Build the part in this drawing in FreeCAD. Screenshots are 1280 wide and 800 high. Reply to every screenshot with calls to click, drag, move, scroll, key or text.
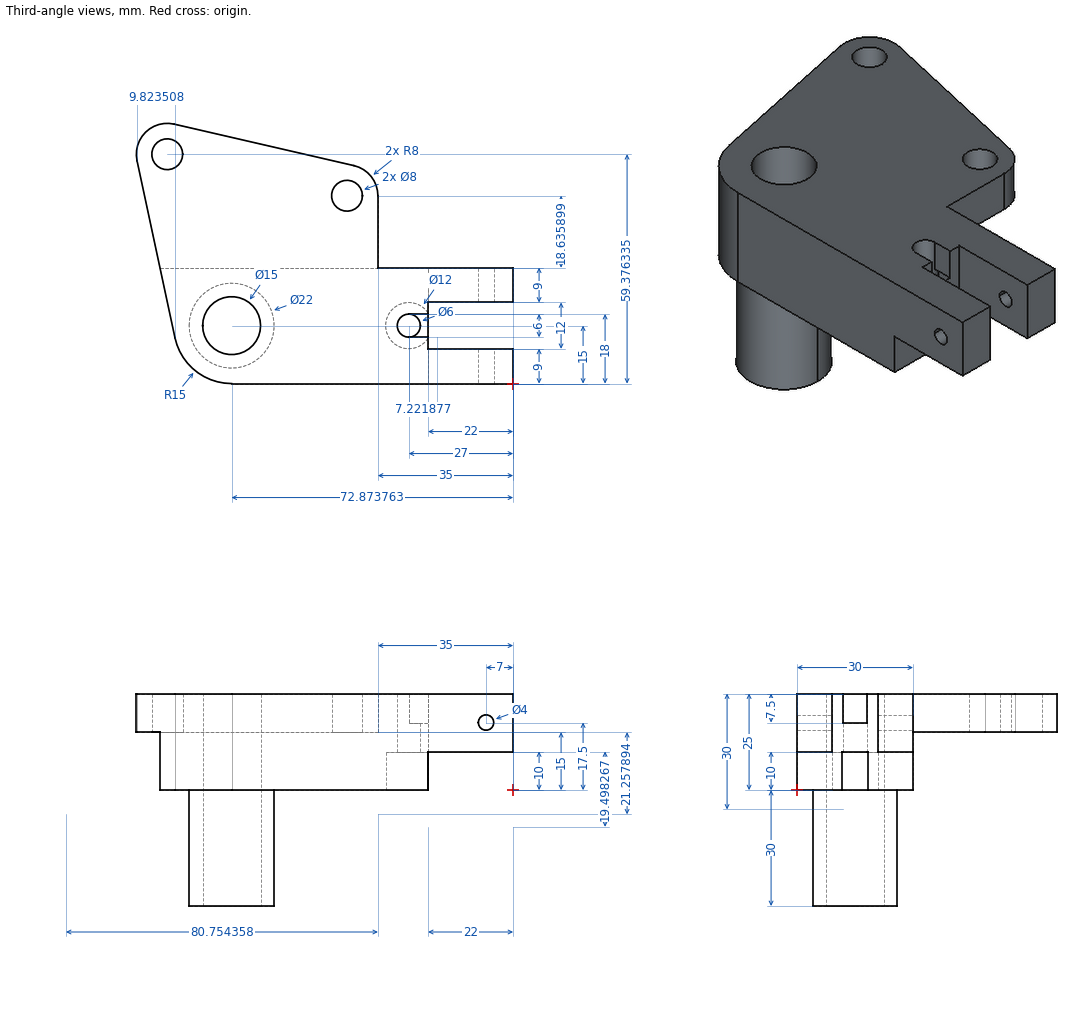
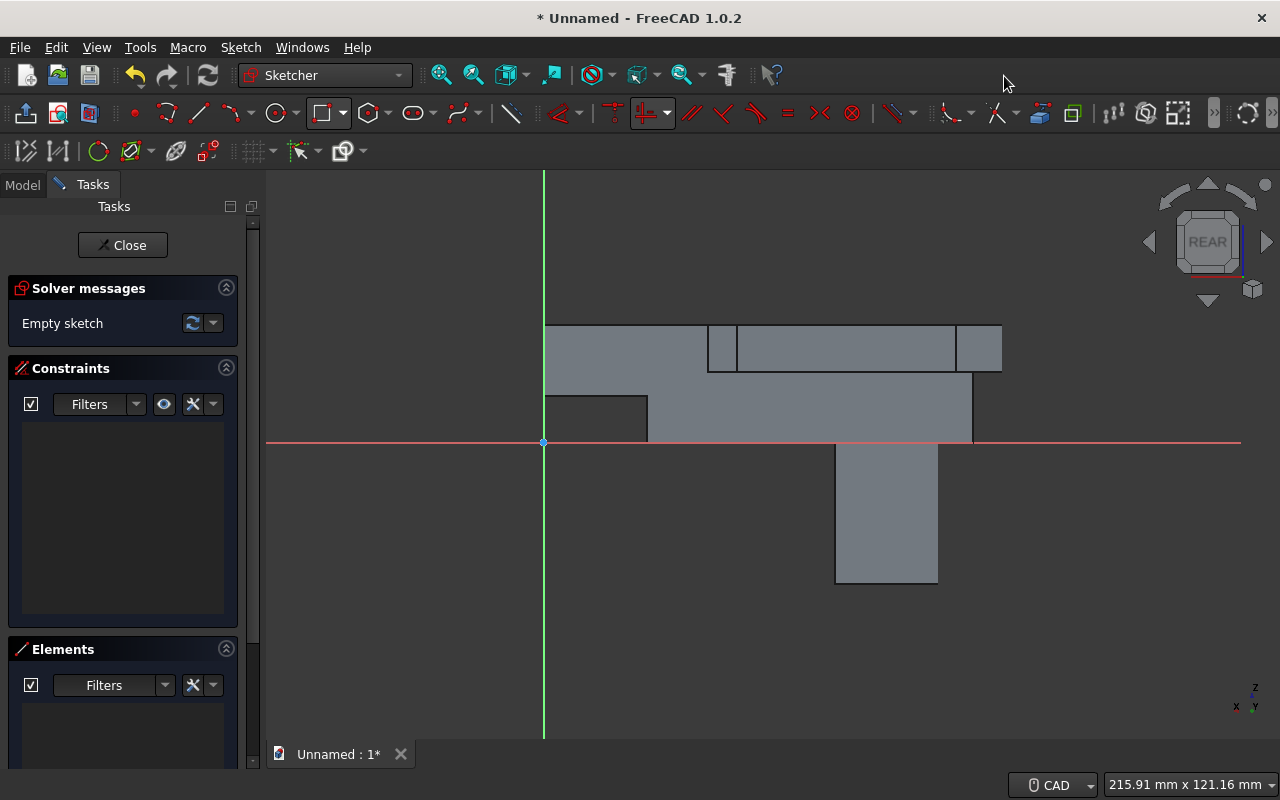
scroll(570, 356, up, 15)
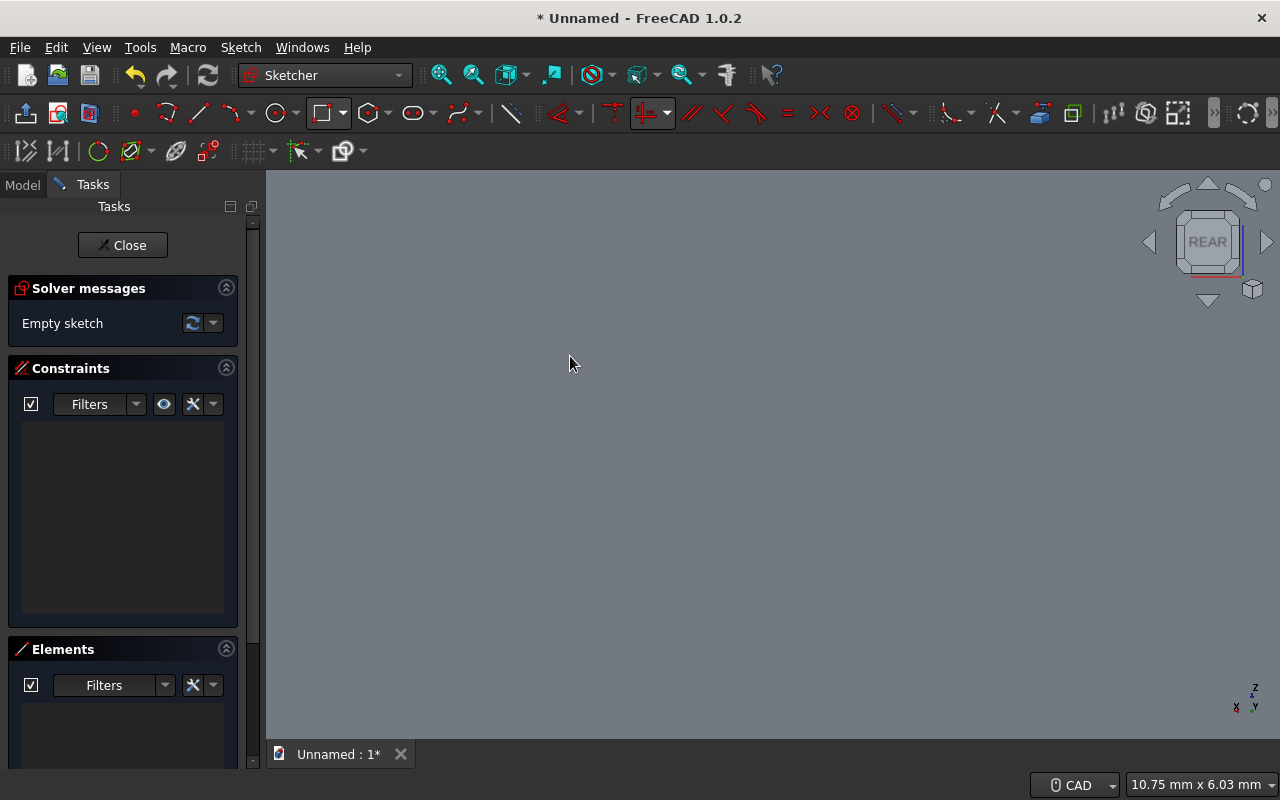
click(276, 114)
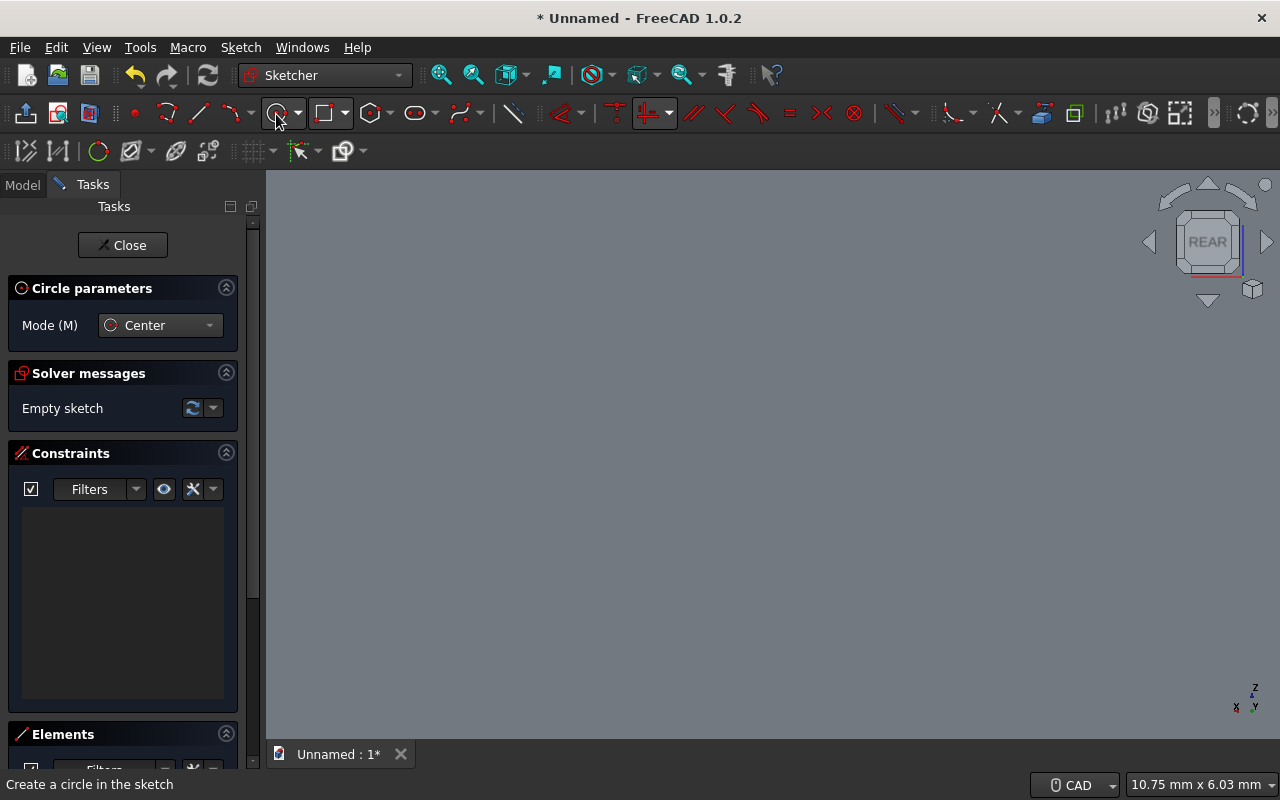
click(701, 442)
click(835, 308)
key(Escape)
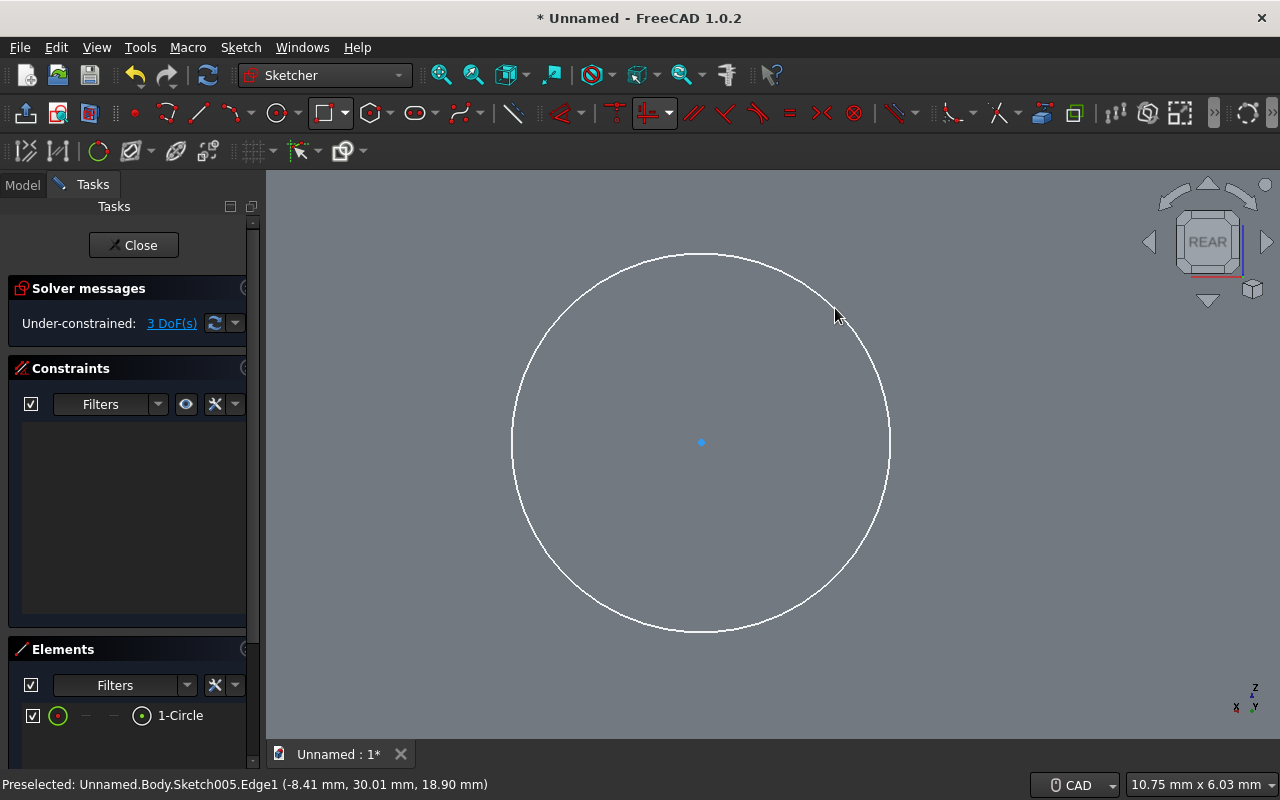
click(560, 114)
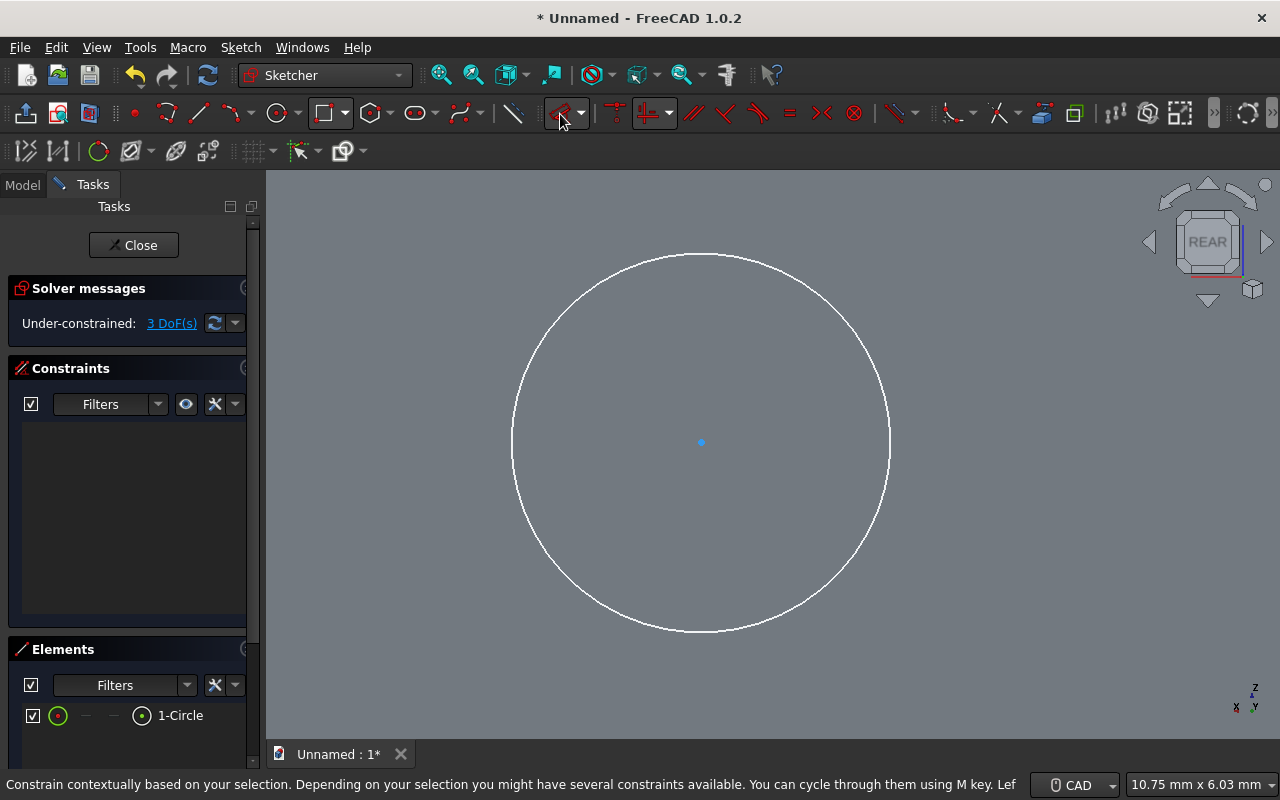
click(835, 309)
click(858, 286)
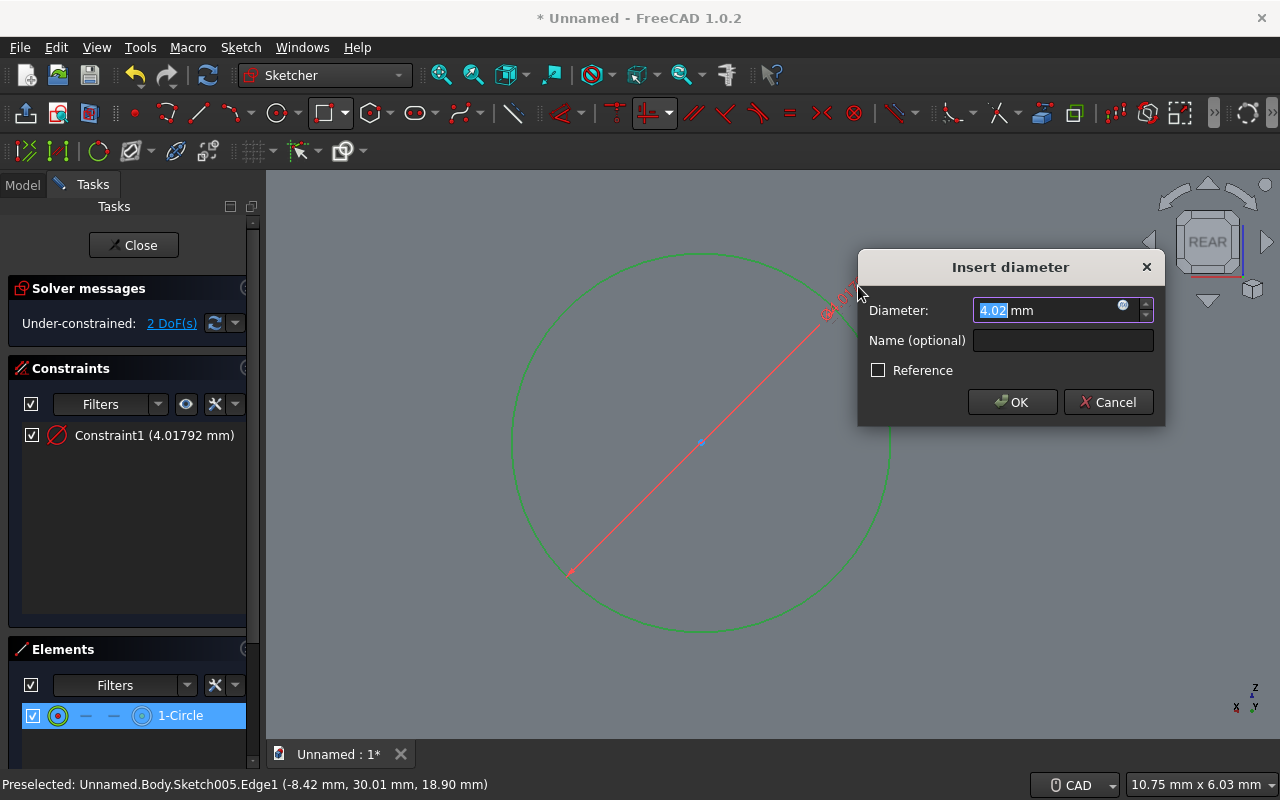
text(4)
key(Return)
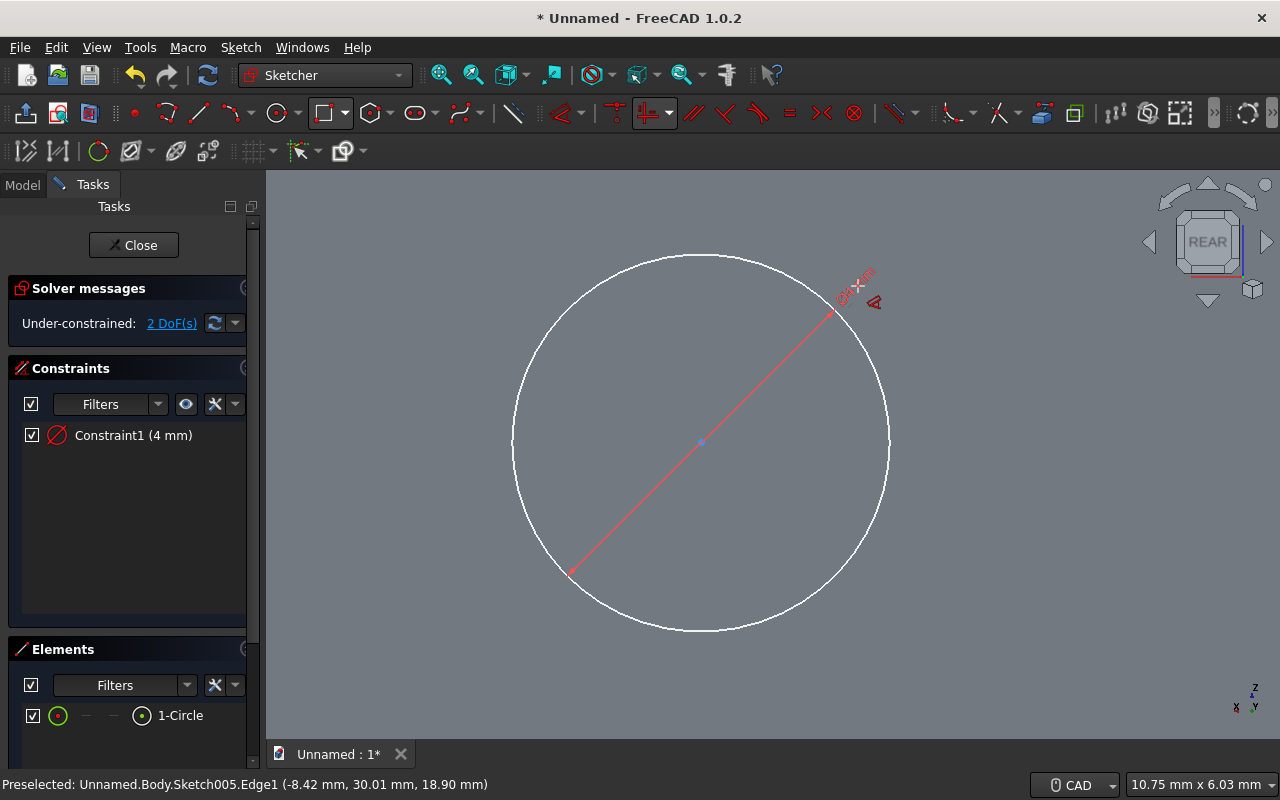
click(701, 443)
click(497, 409)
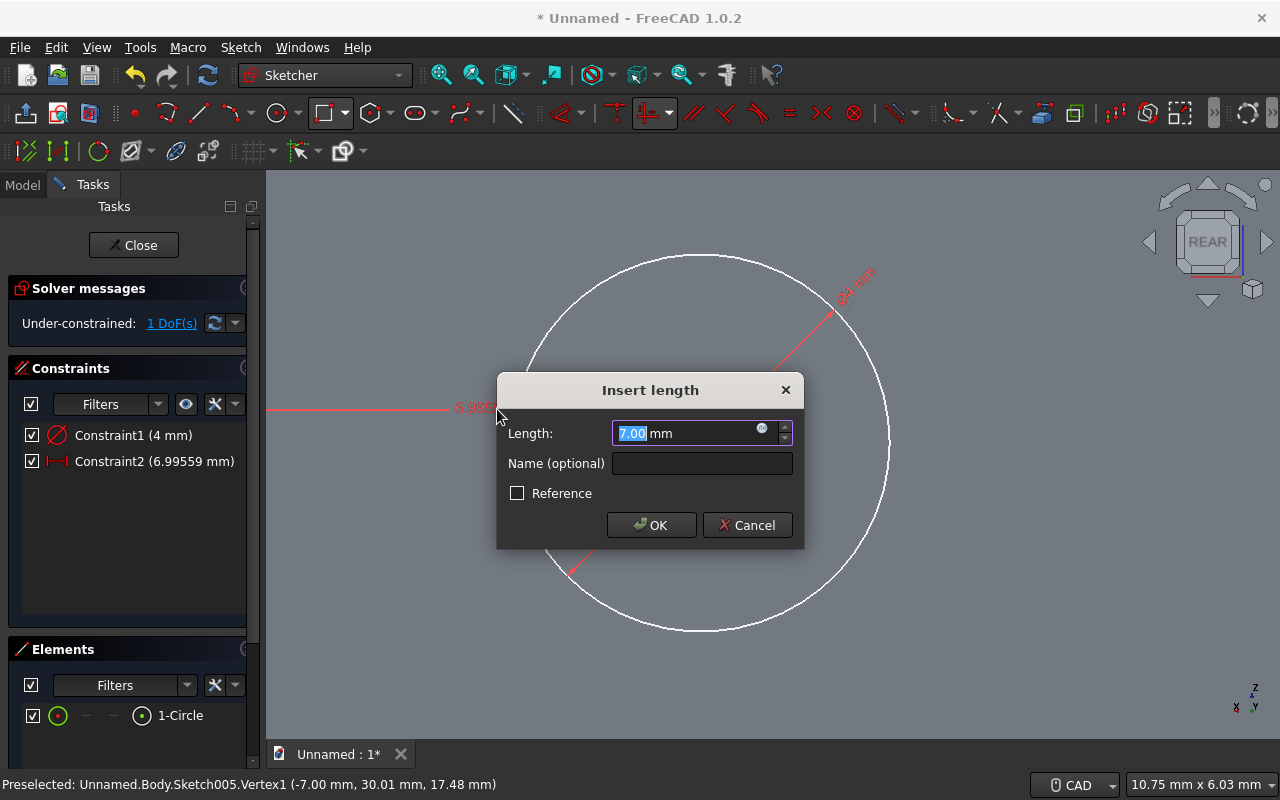
text(7)
key(Return)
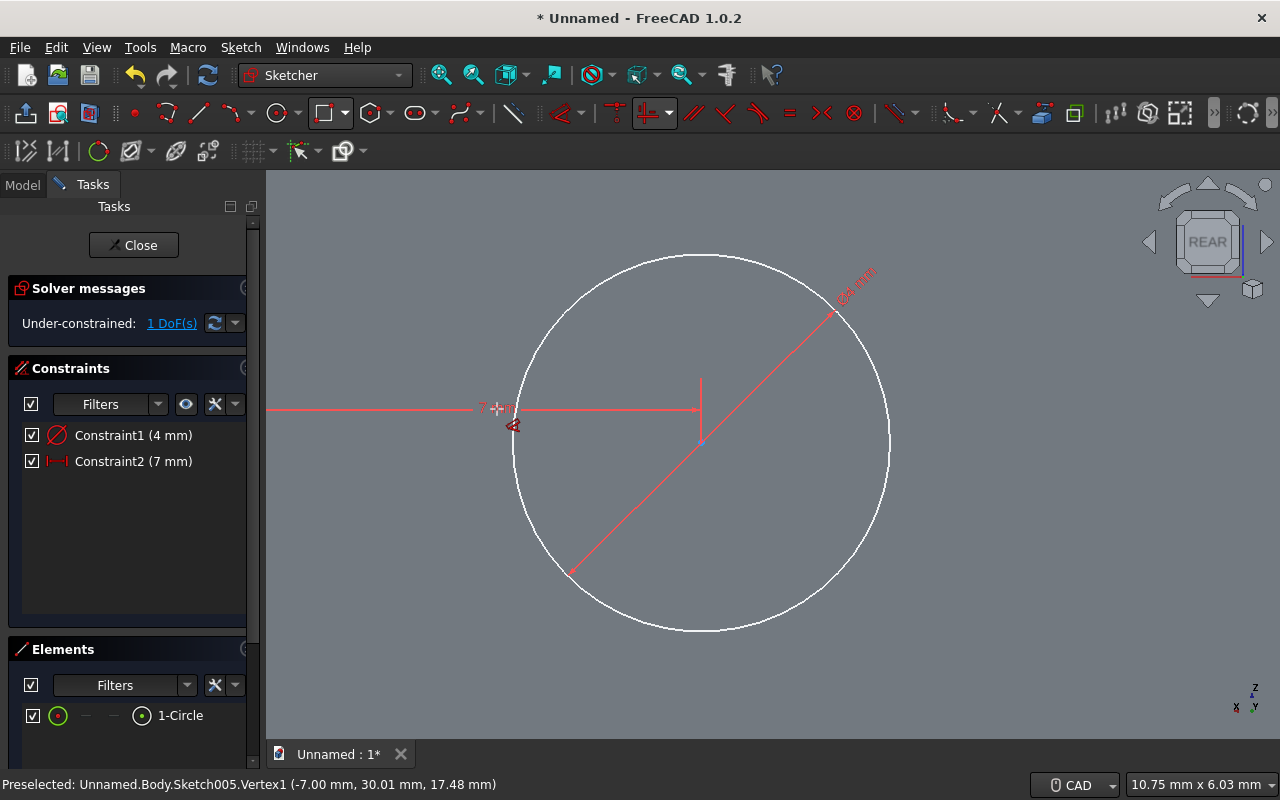
click(701, 443)
click(735, 577)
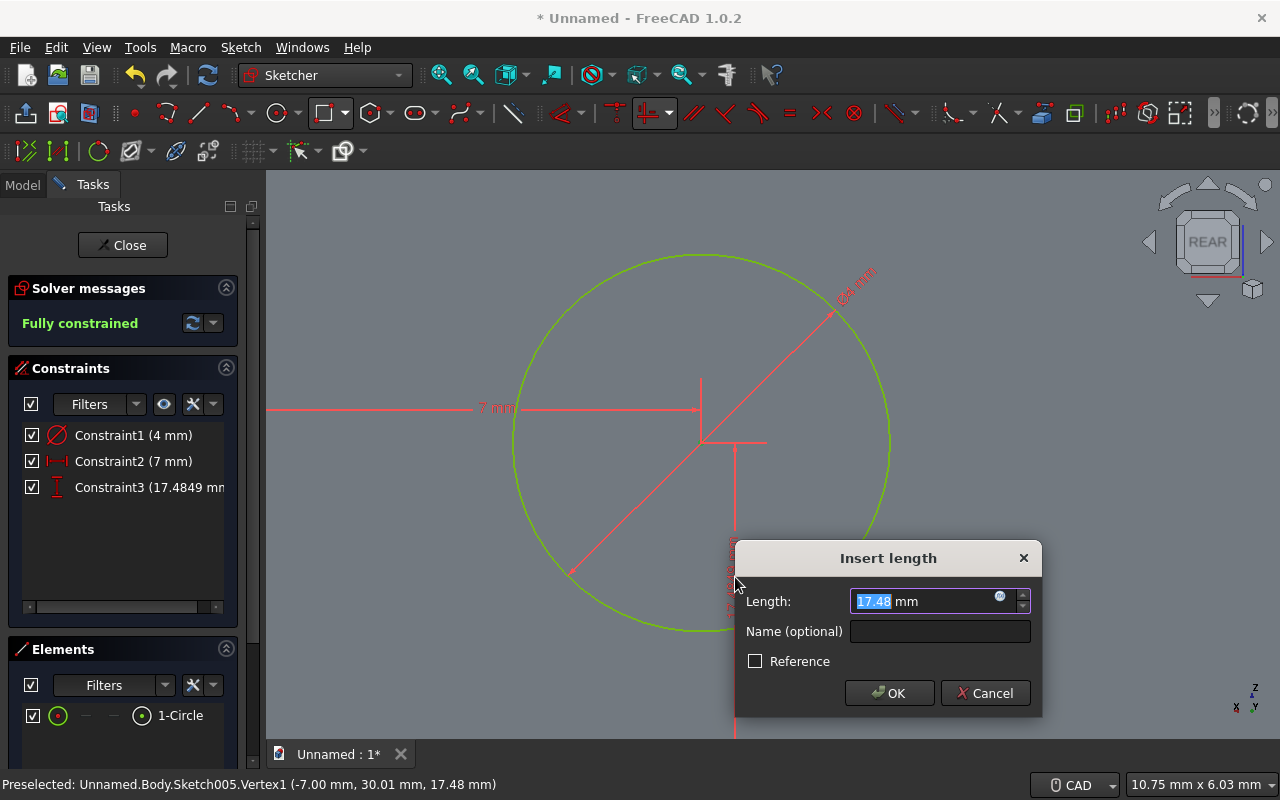
text(17.5)
key(Return)
key(Escape)